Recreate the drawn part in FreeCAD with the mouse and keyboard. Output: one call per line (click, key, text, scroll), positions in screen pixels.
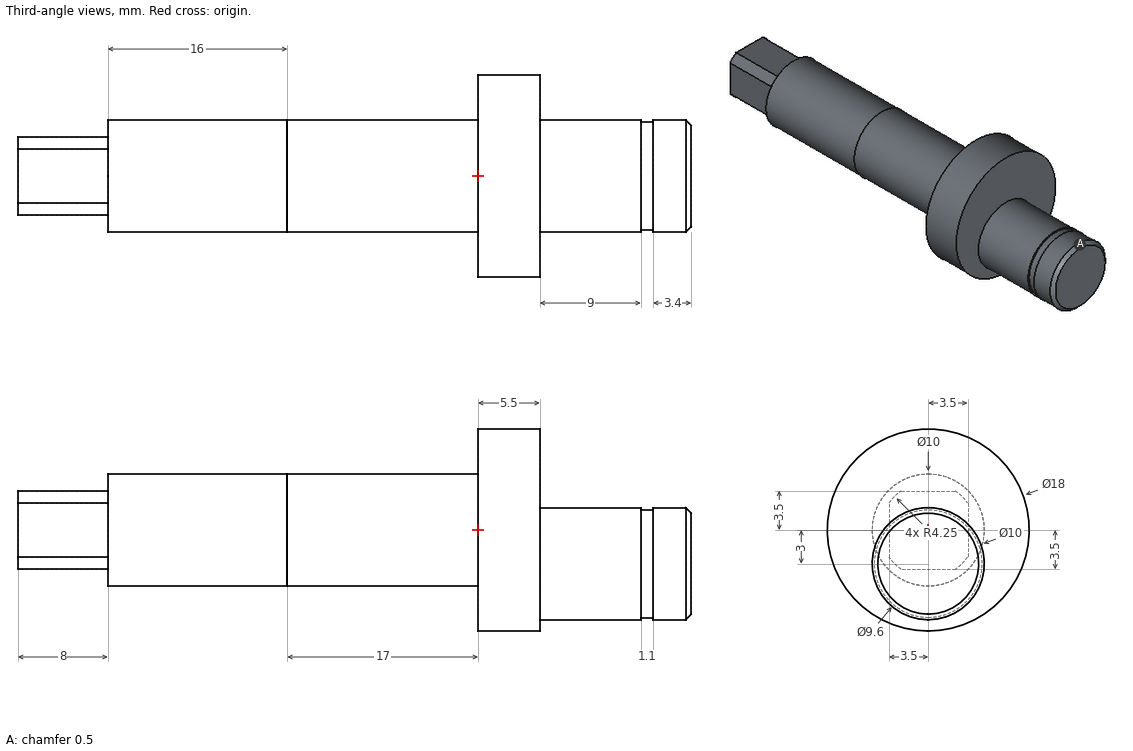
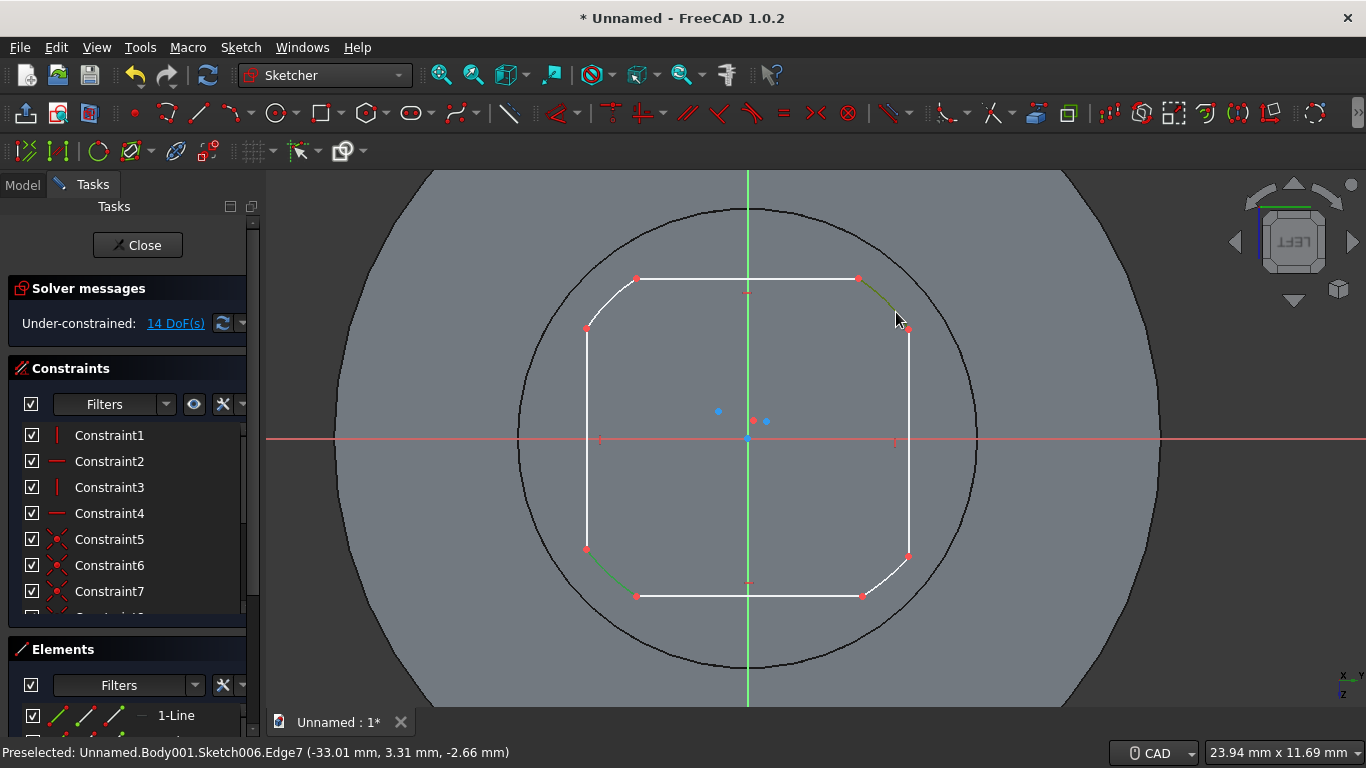
key(c)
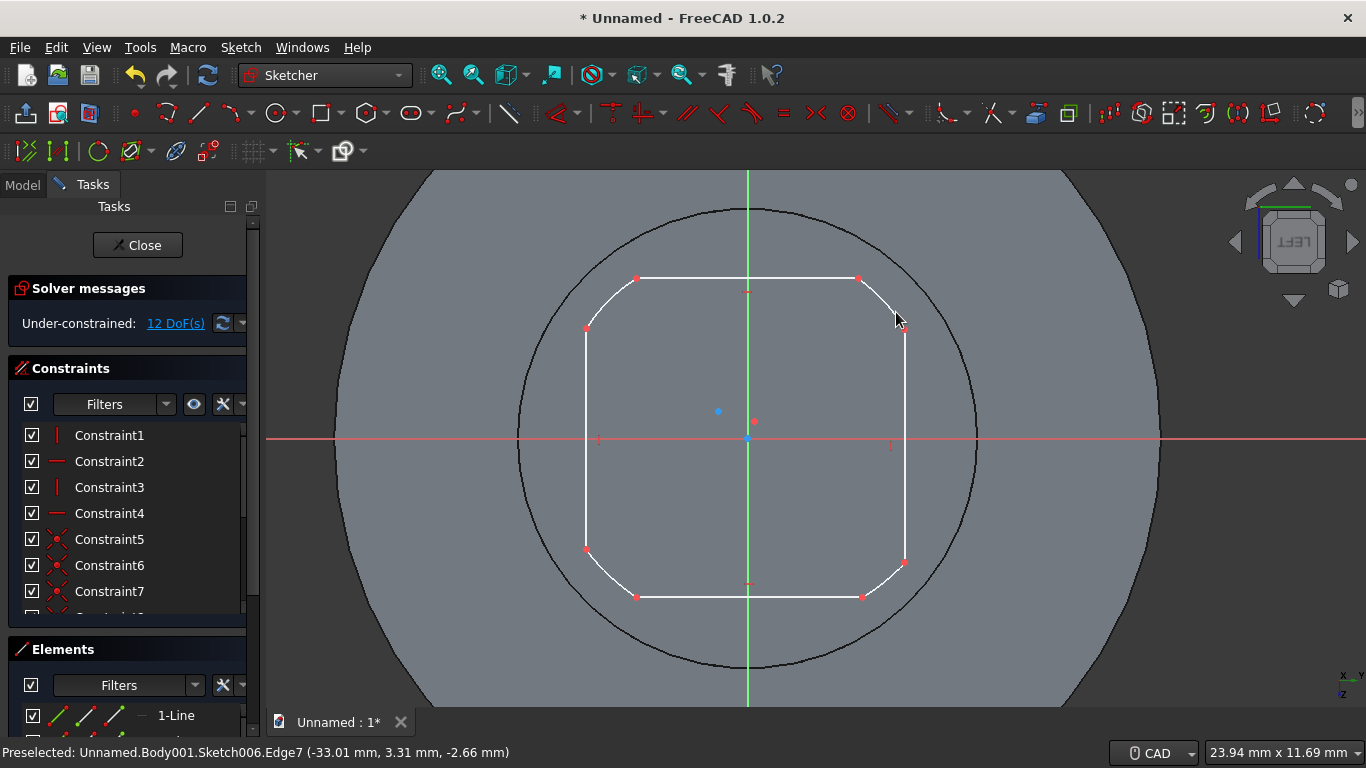
click(600, 566)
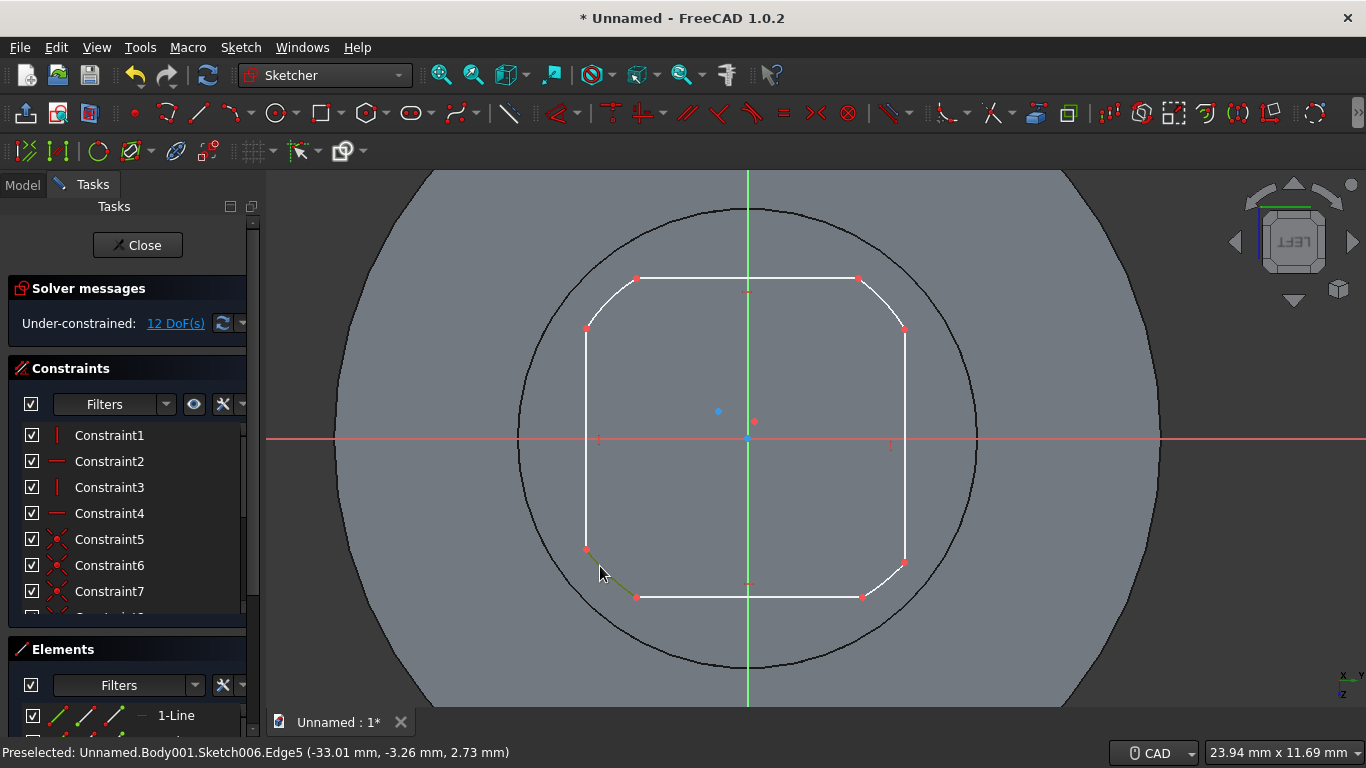
click(619, 291)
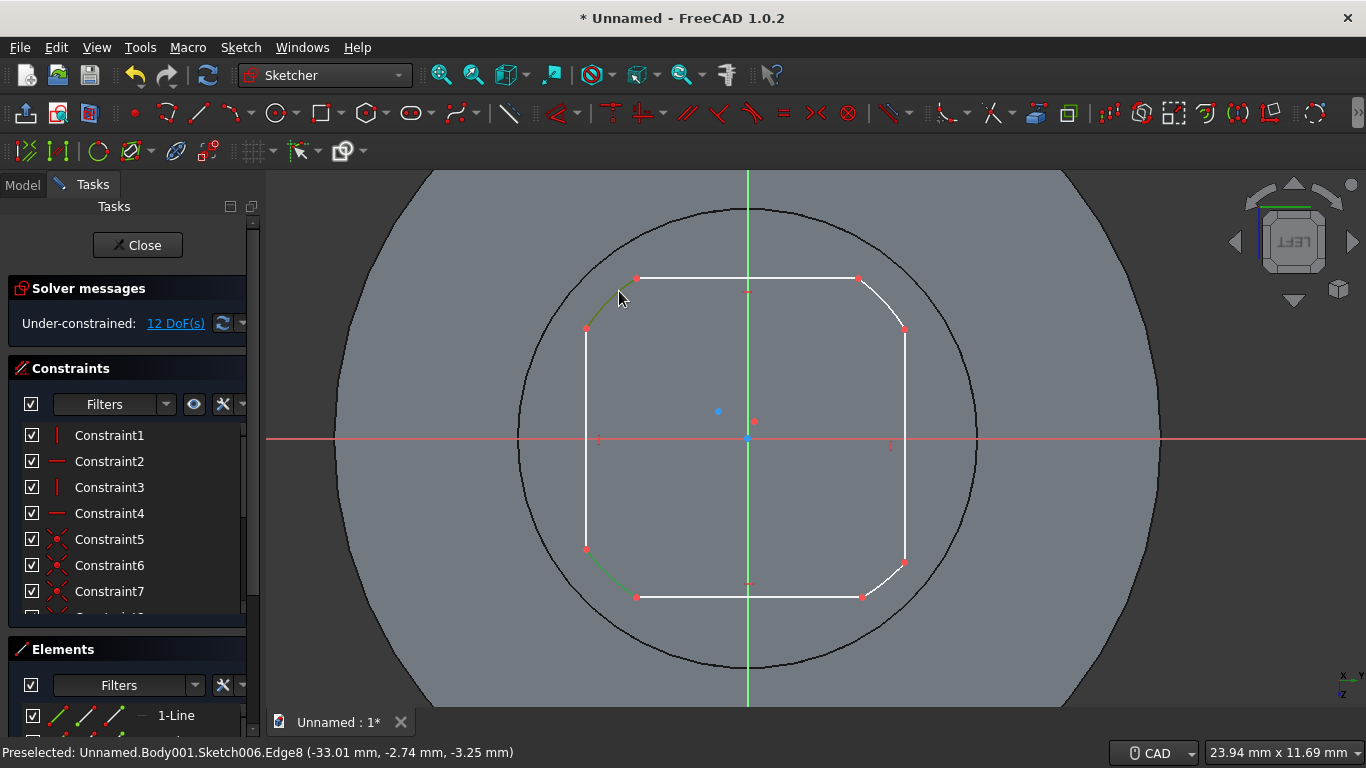
click(612, 114)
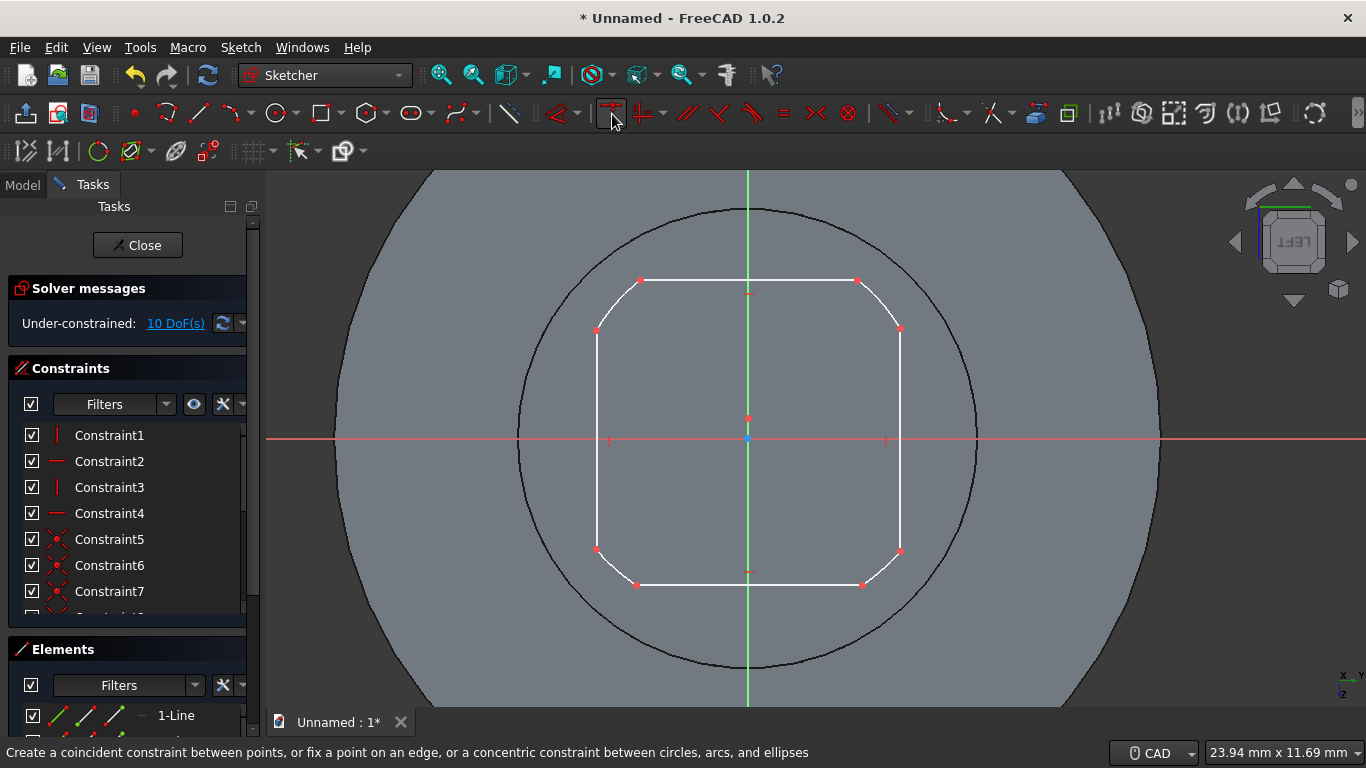
drag(738, 409, 758, 449)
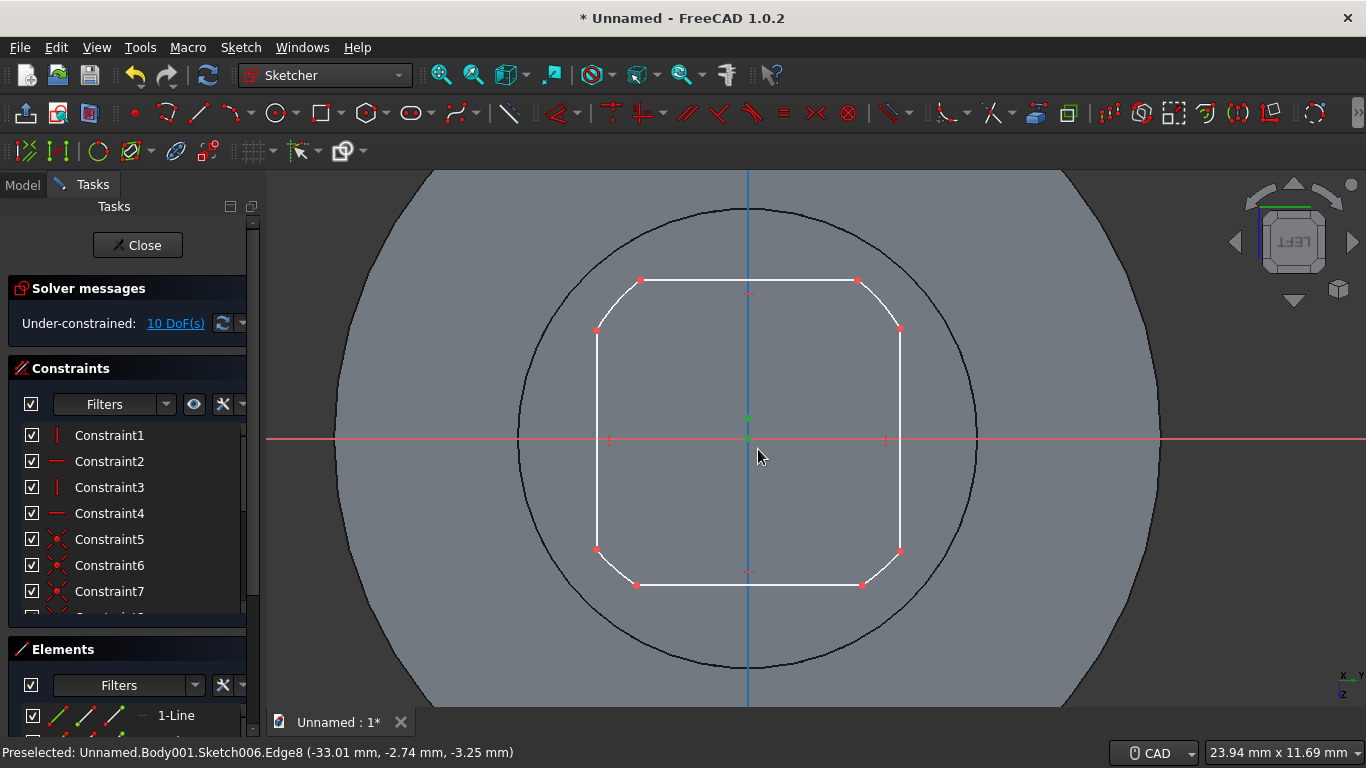
key(c)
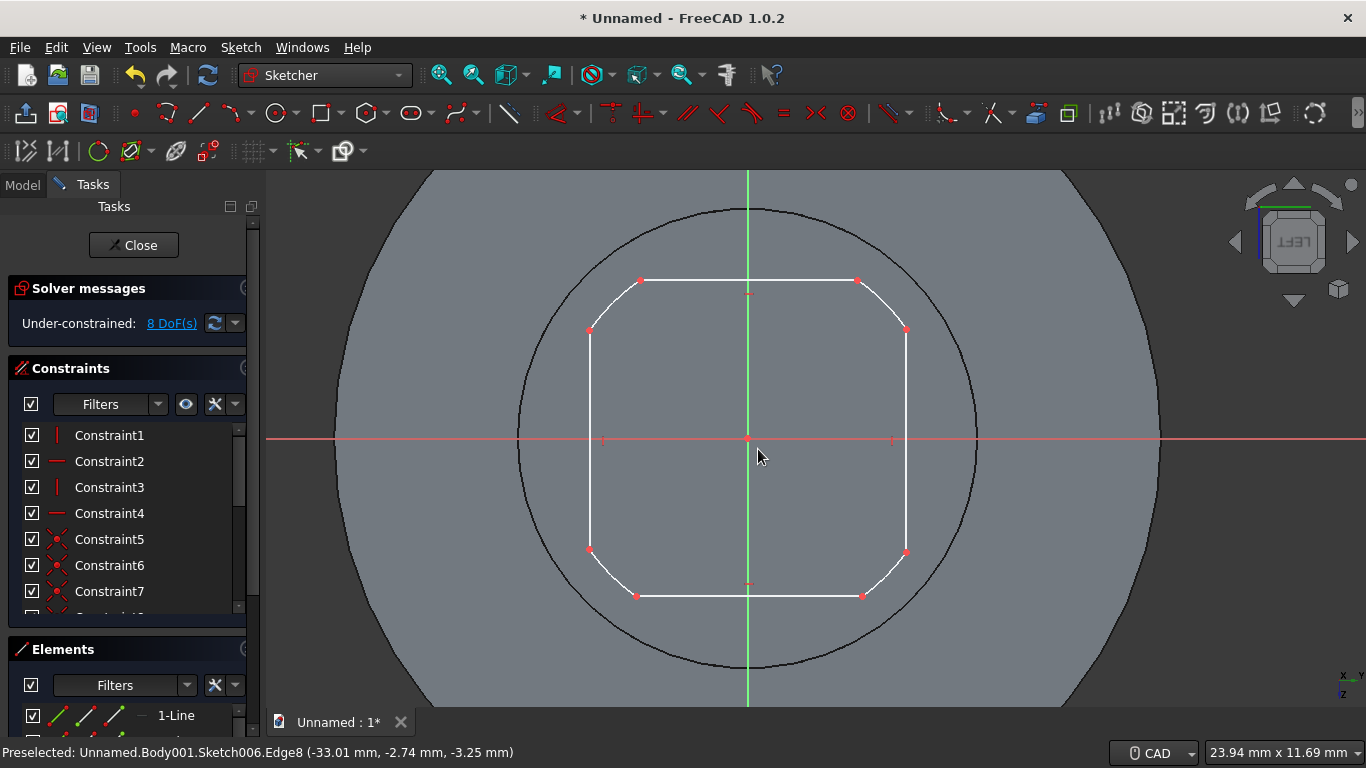
click(602, 566)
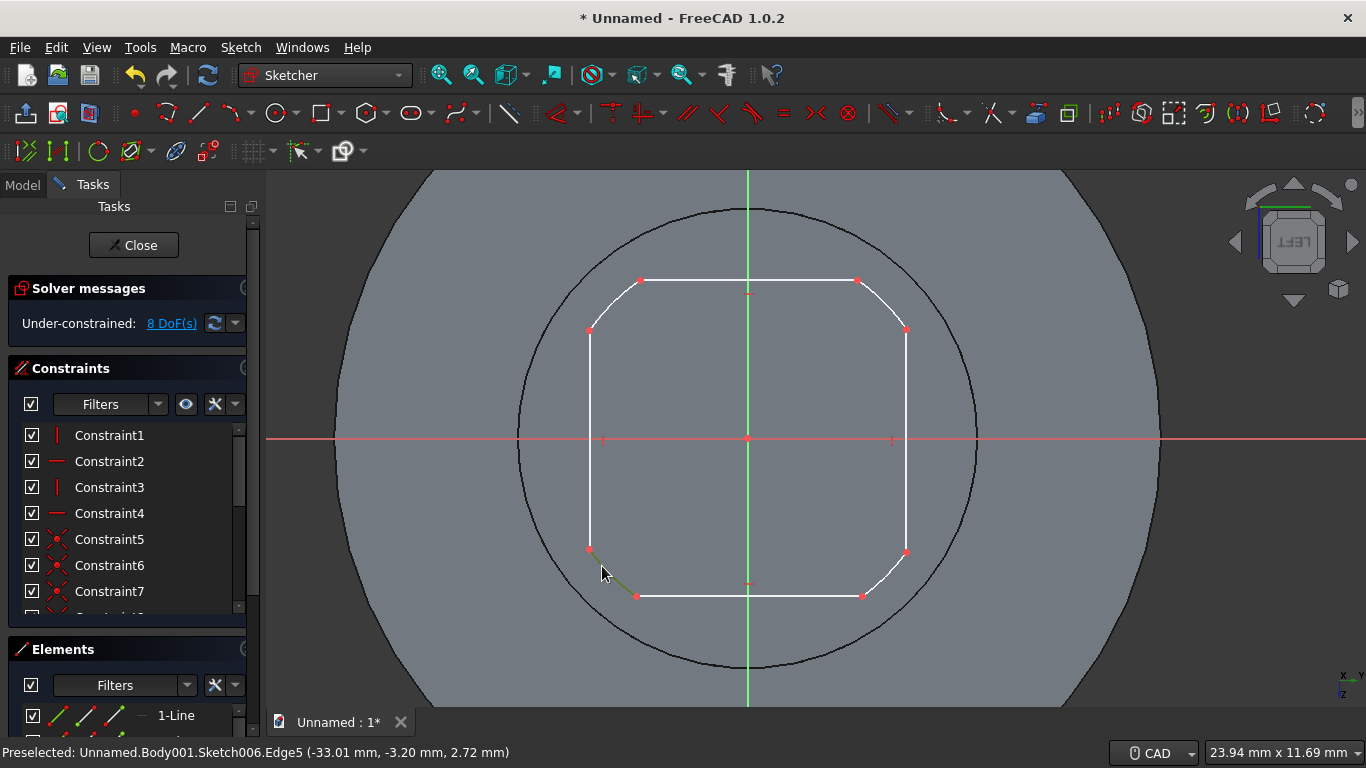
click(877, 585)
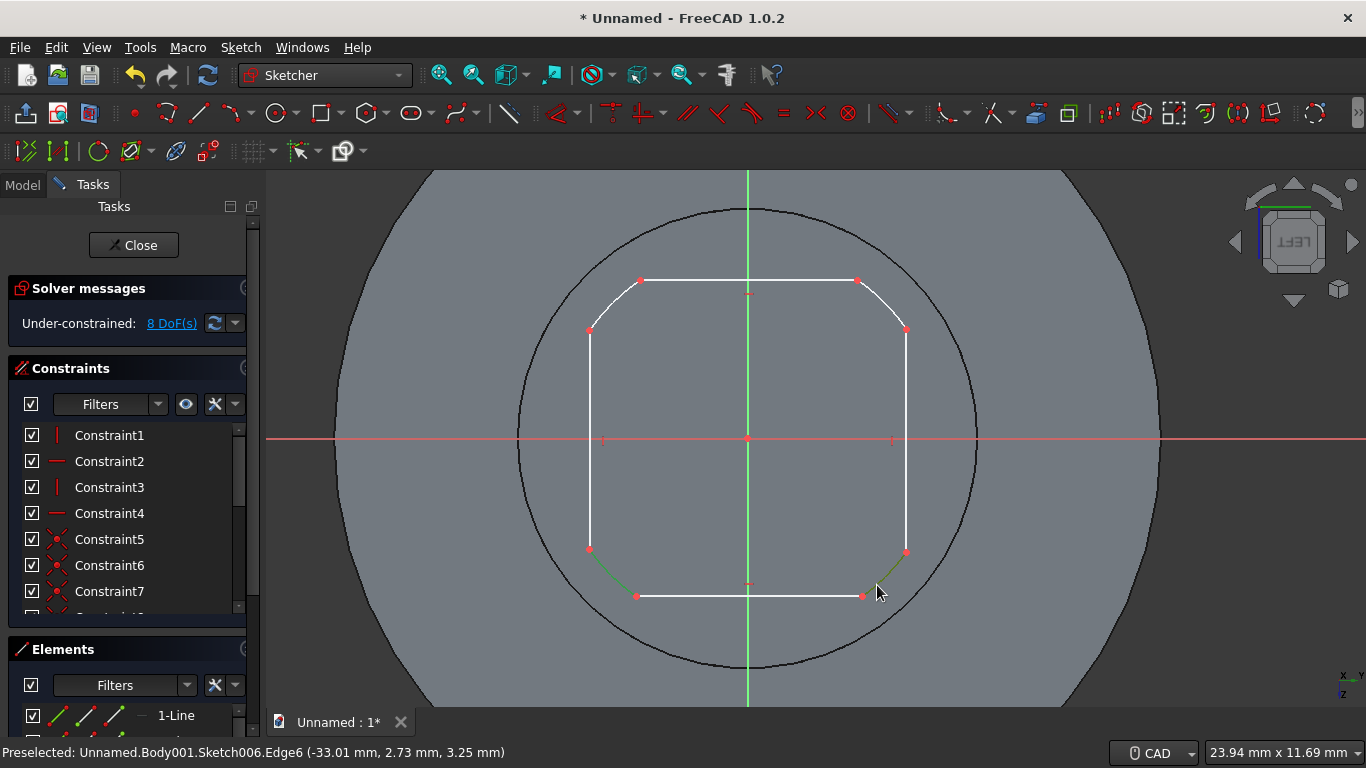
click(894, 313)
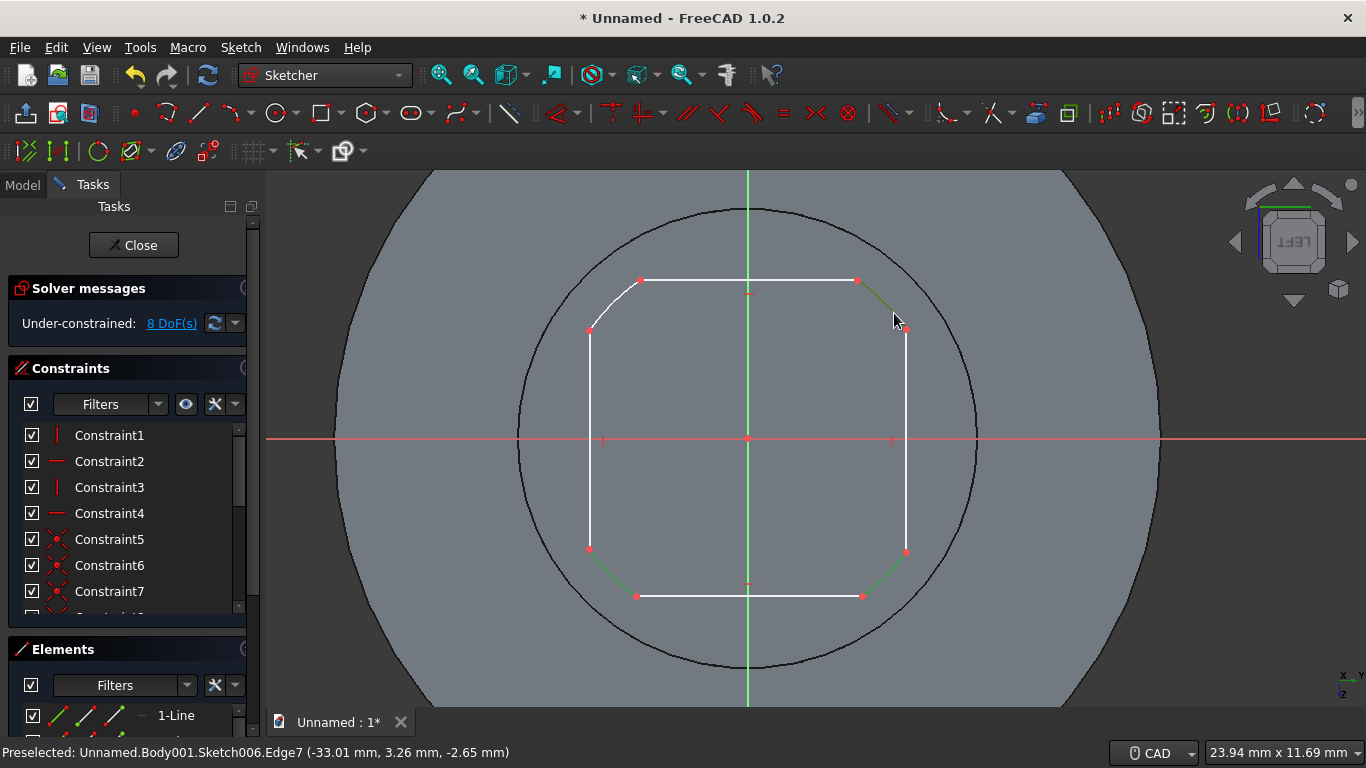
click(623, 293)